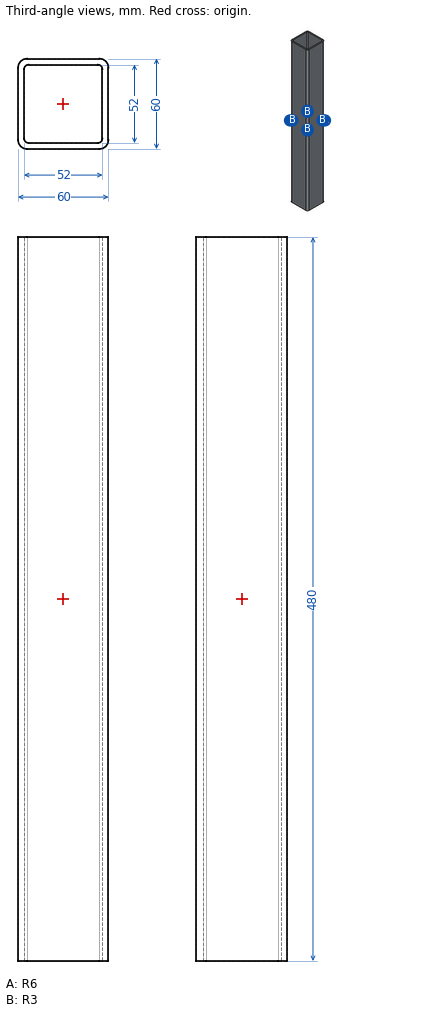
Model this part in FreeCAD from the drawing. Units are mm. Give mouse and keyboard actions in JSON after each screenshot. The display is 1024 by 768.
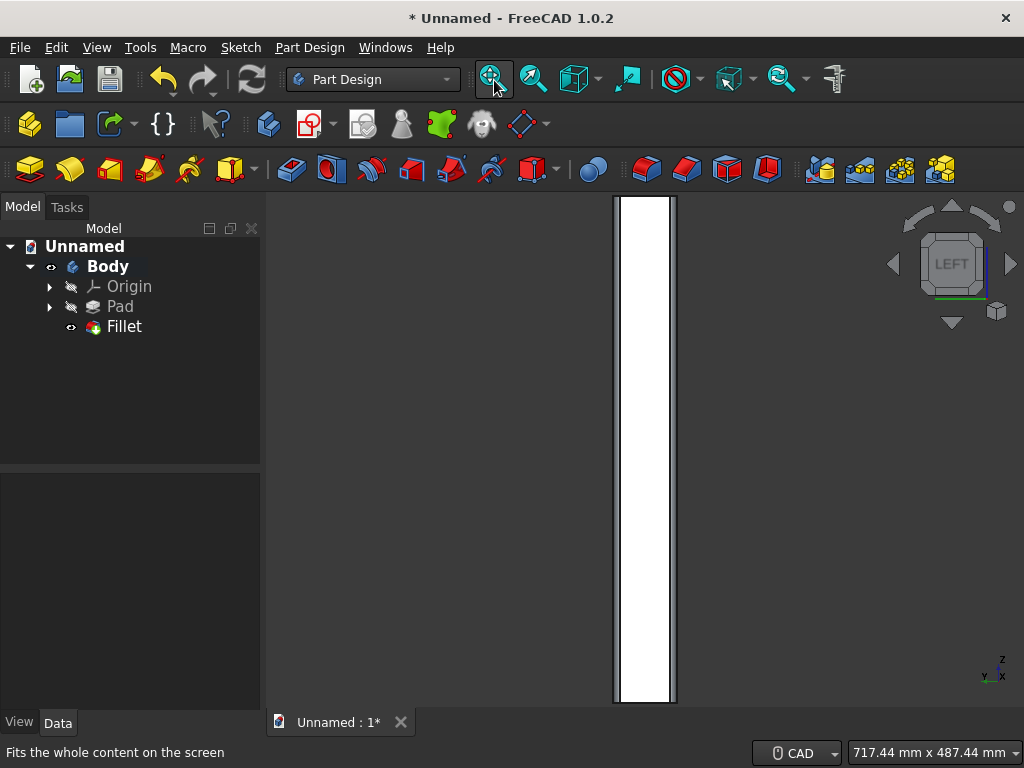
{"action": "key", "text": "v 3"}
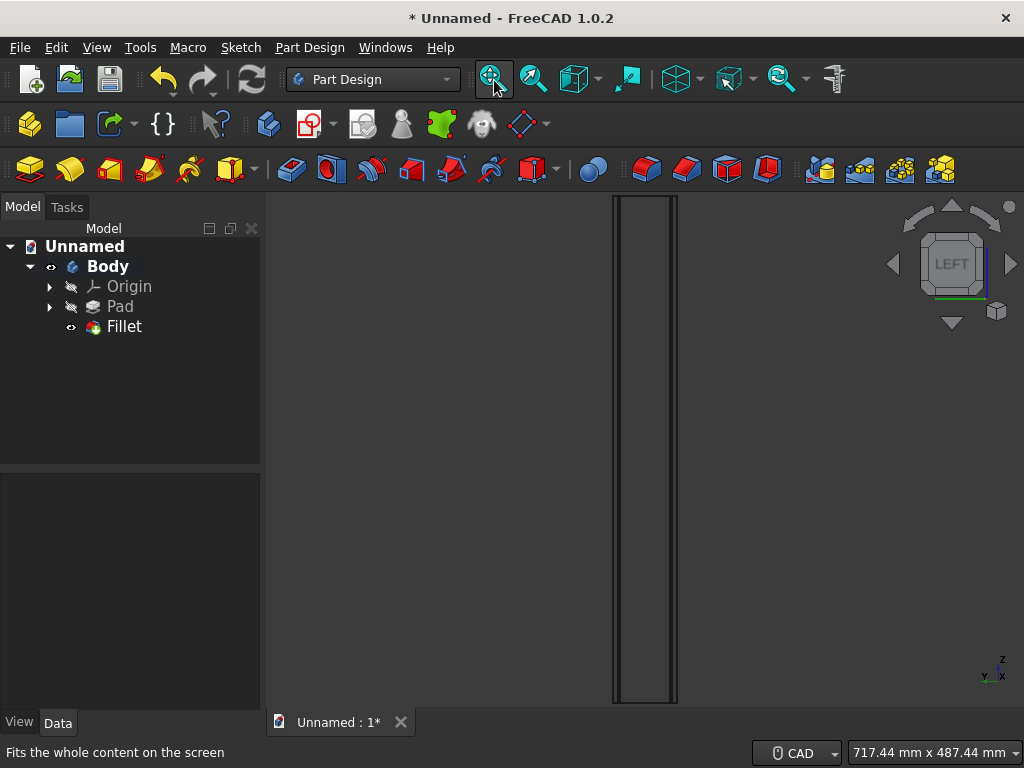
{"action": "key", "text": "0"}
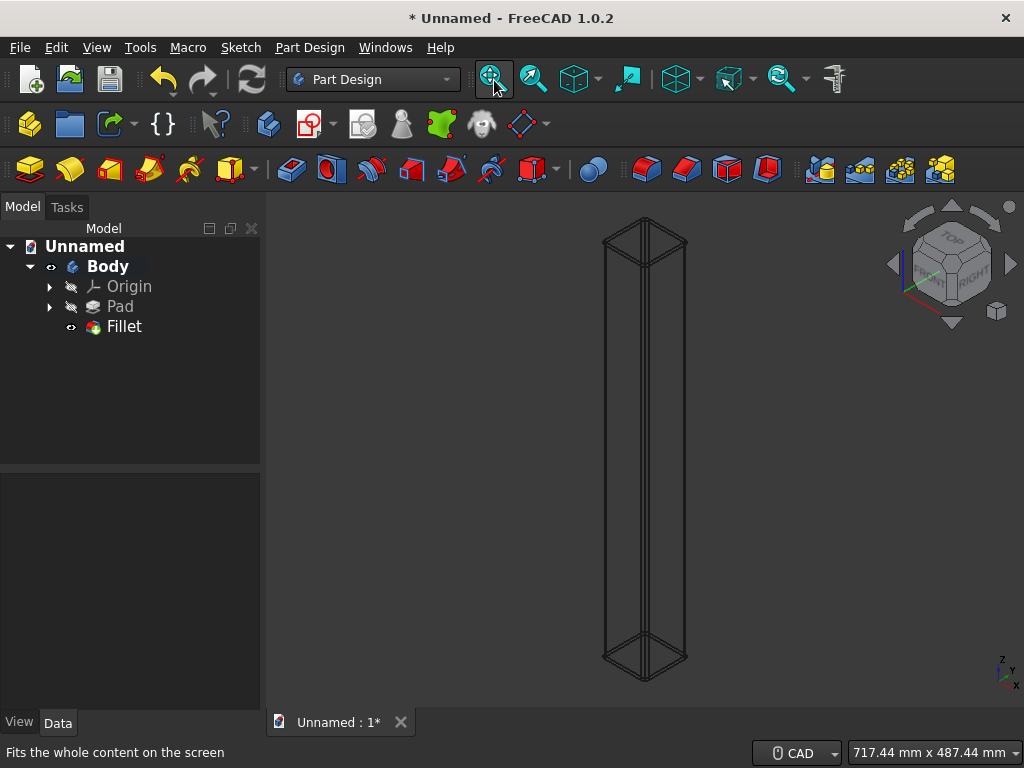
{"action": "scroll", "coordinate": [645, 471], "scroll_direction": "up", "scroll_amount": 6}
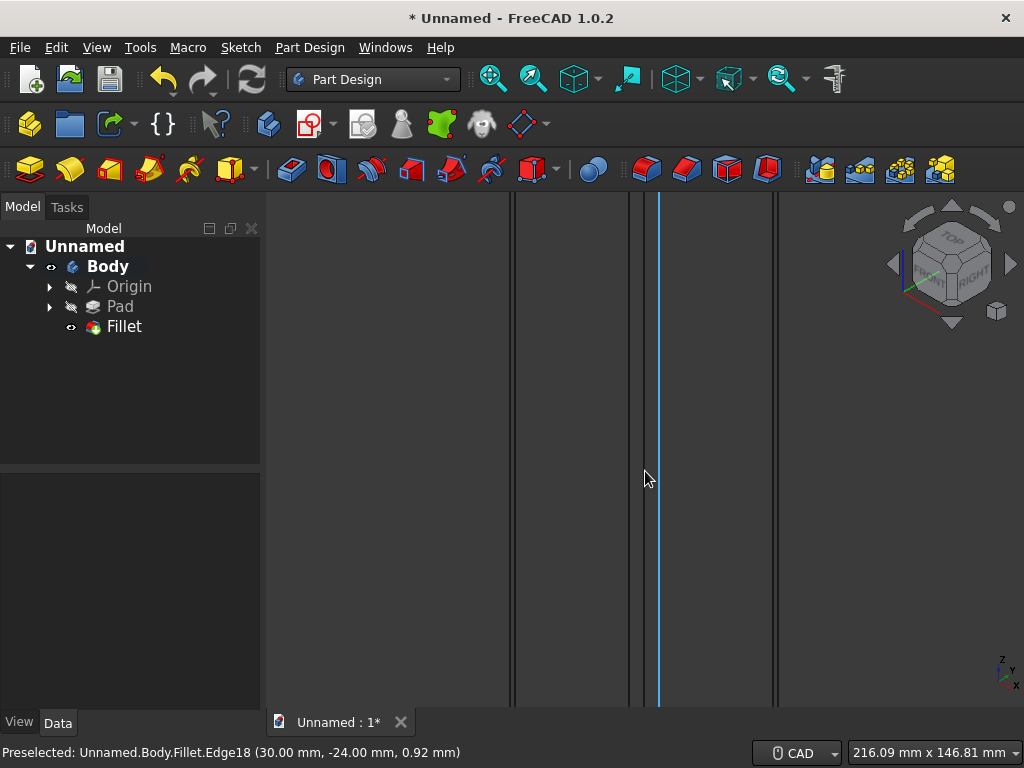
{"action": "left_click", "coordinate": [644, 472]}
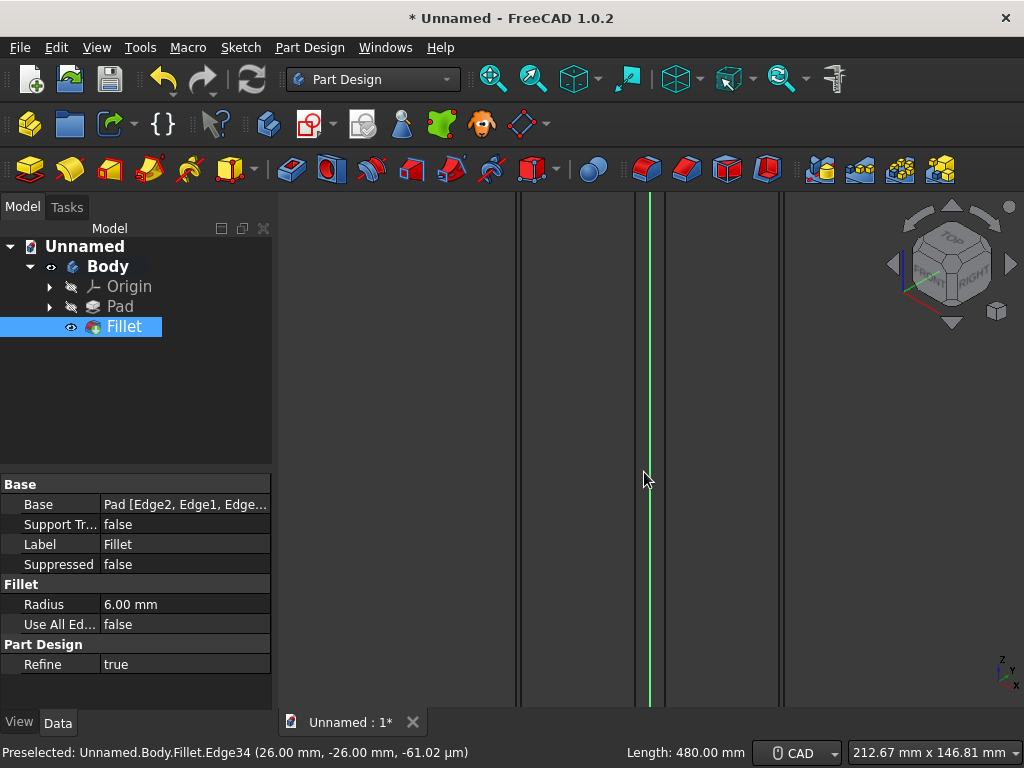
{"action": "left_click", "coordinate": [494, 80]}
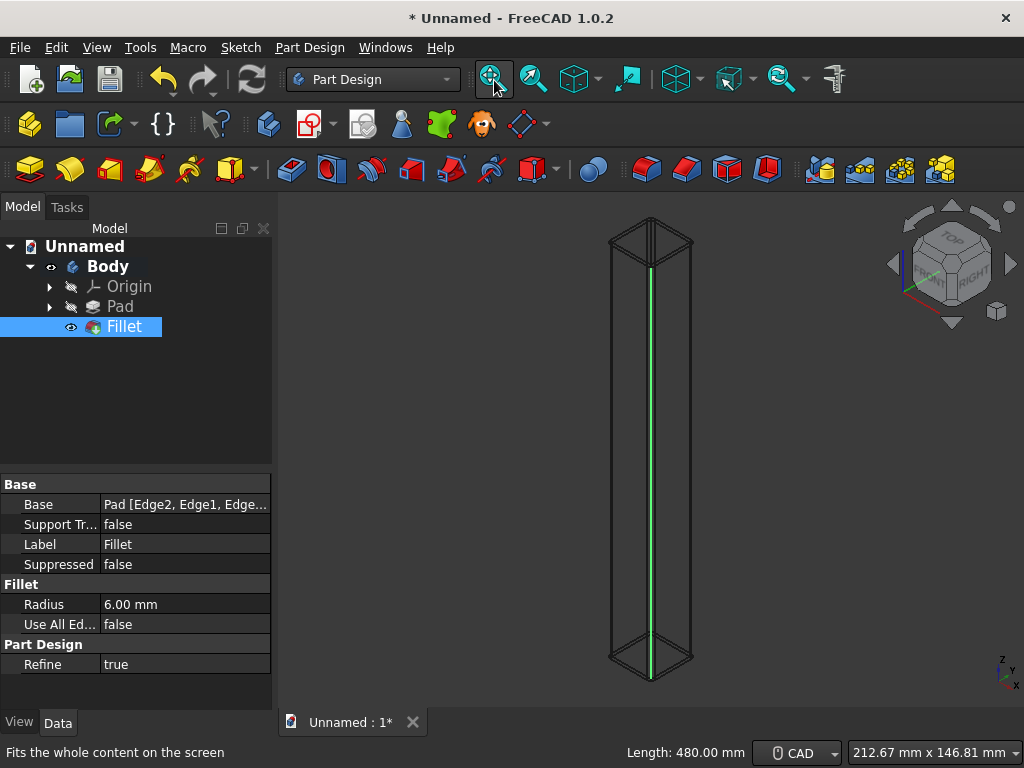
{"action": "key", "text": "2"}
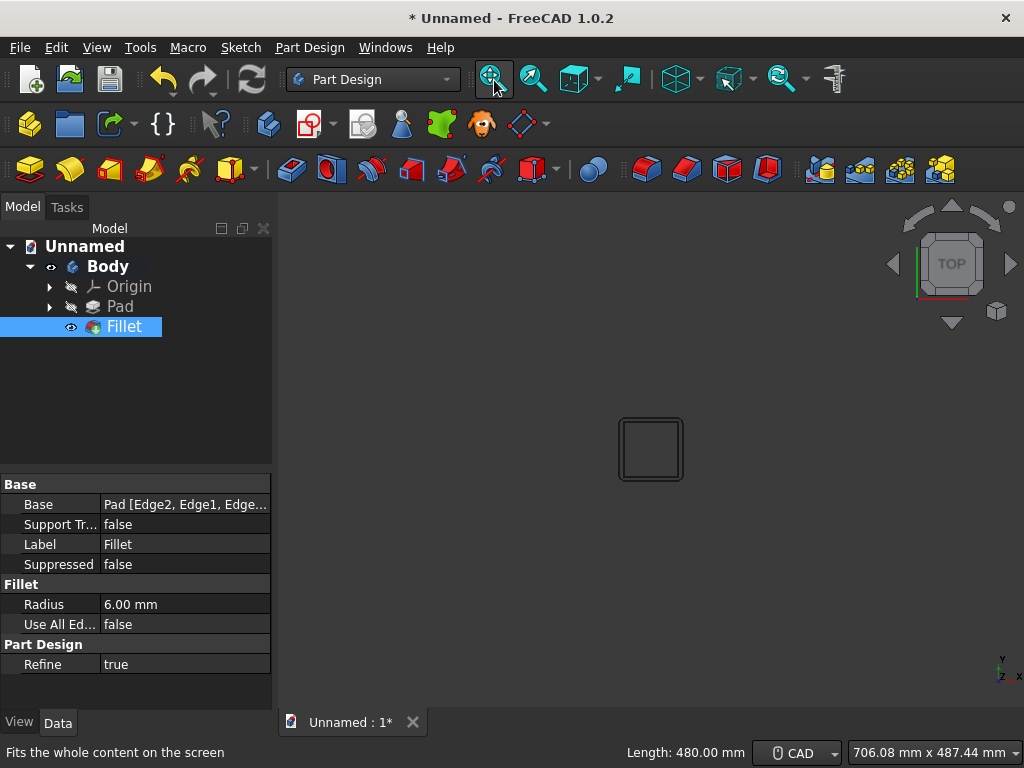
{"action": "left_click", "coordinate": [494, 80]}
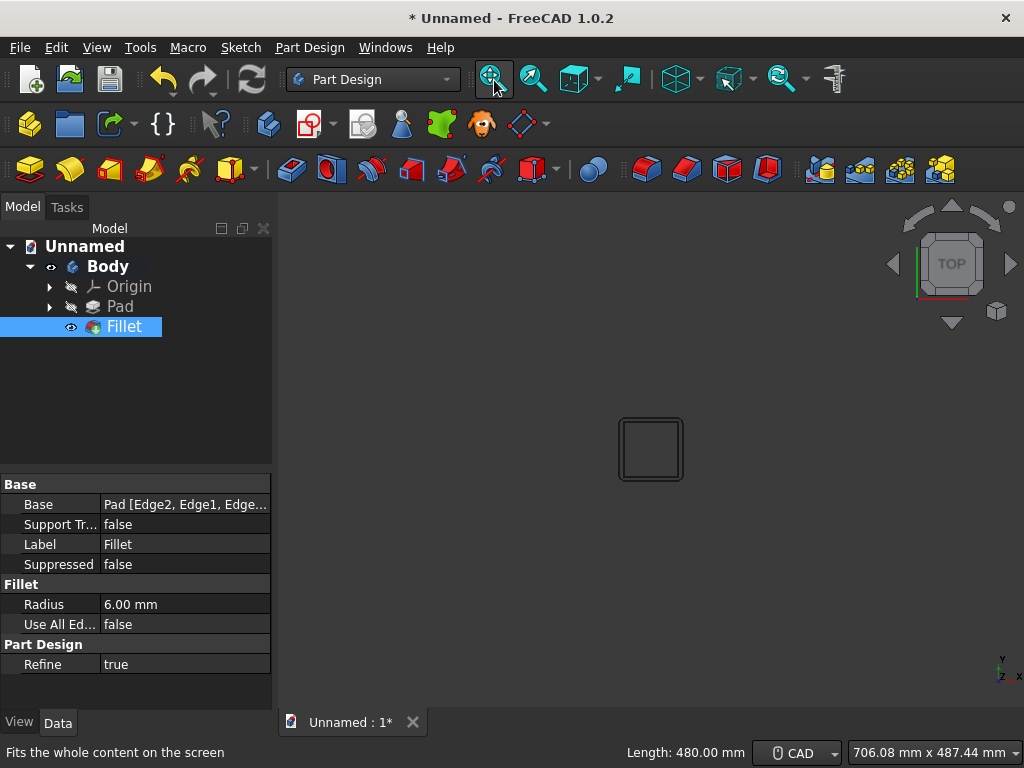
{"action": "scroll", "coordinate": [678, 421], "scroll_direction": "up", "scroll_amount": 6}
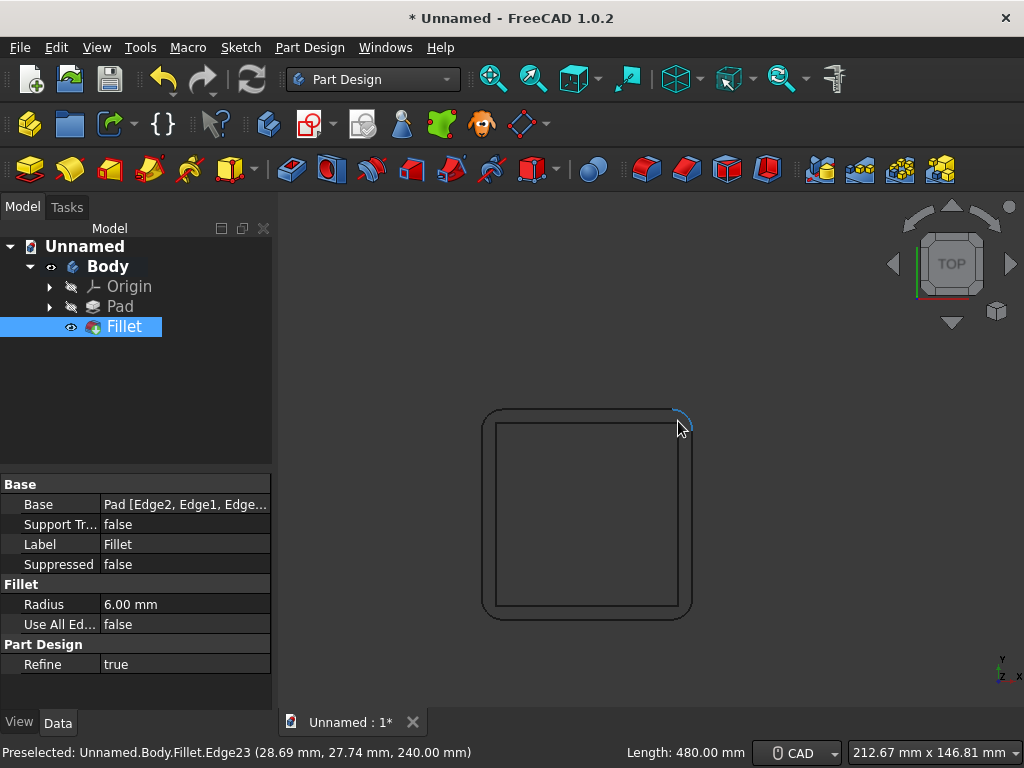
{"action": "left_click", "coordinate": [494, 80]}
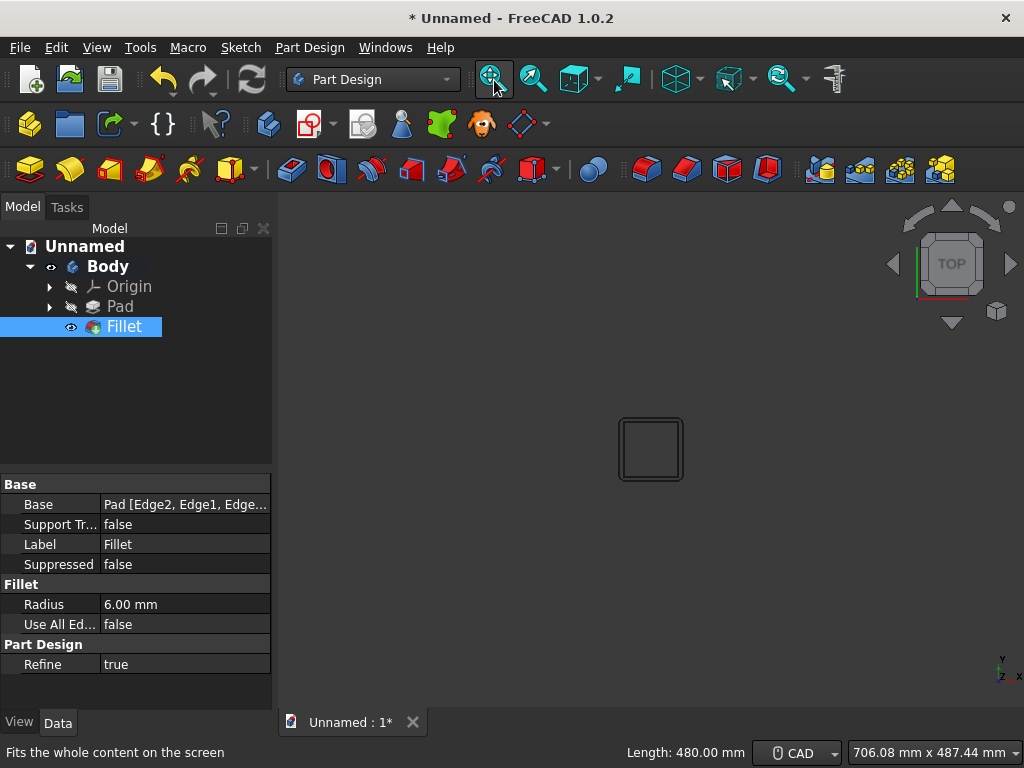
{"action": "key", "text": "1"}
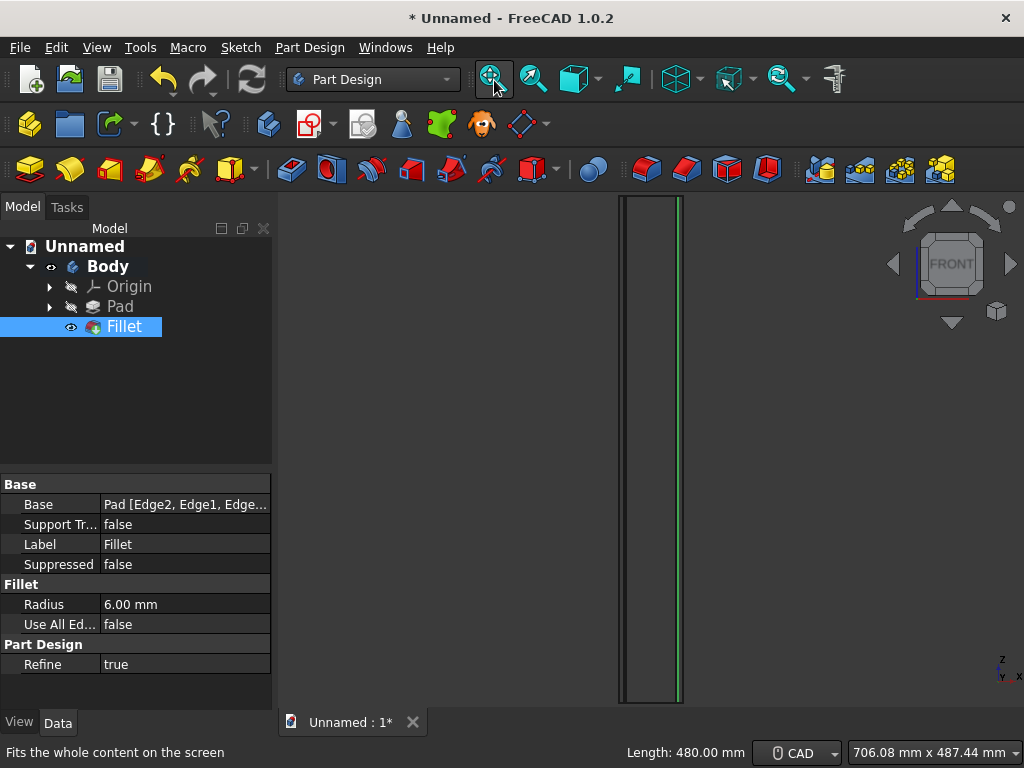
{"action": "scroll", "coordinate": [678, 449], "scroll_direction": "up", "scroll_amount": 6}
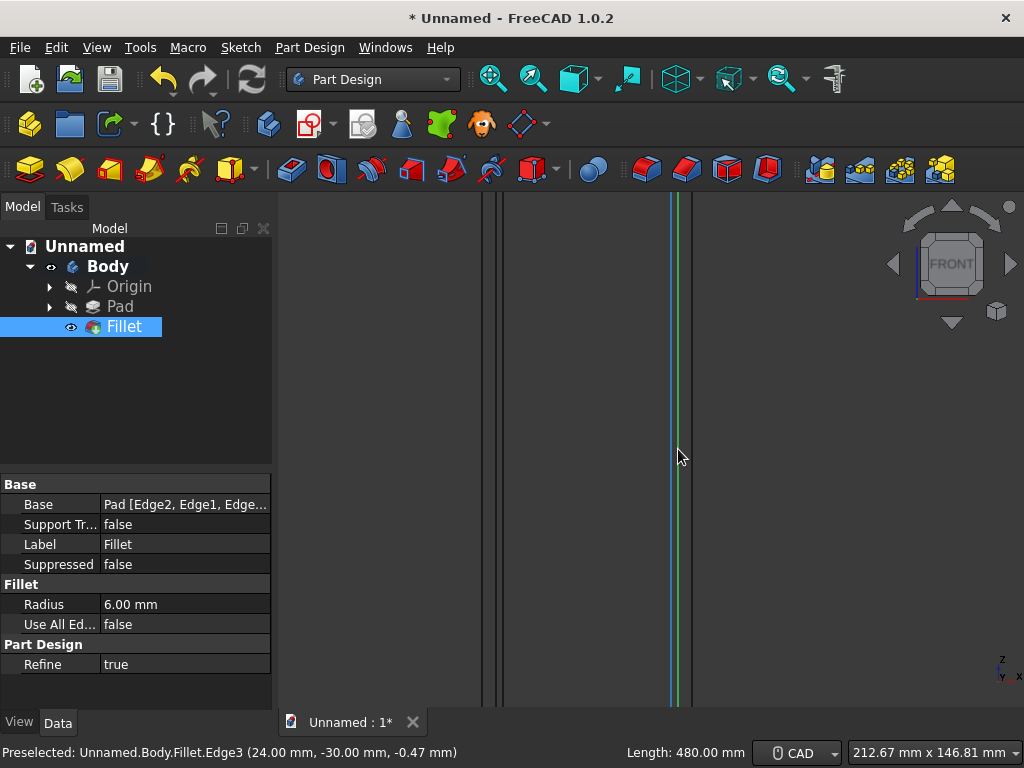
{"action": "left_click", "coordinate": [496, 449], "text": "ctrl"}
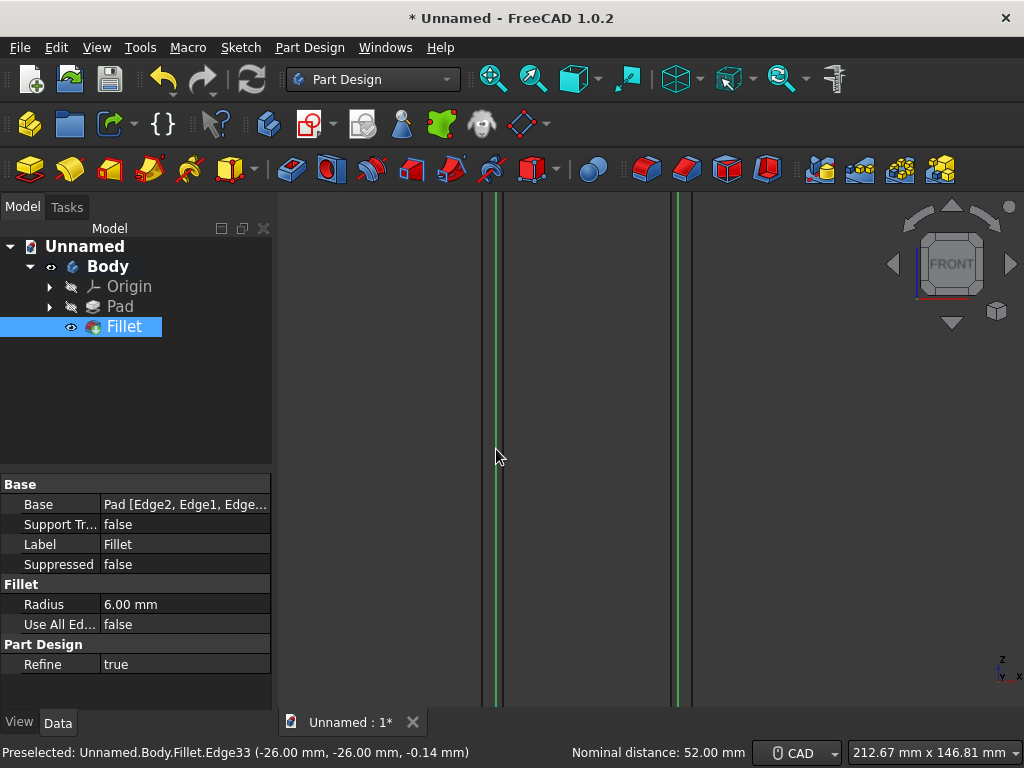
{"action": "left_click", "coordinate": [494, 80]}